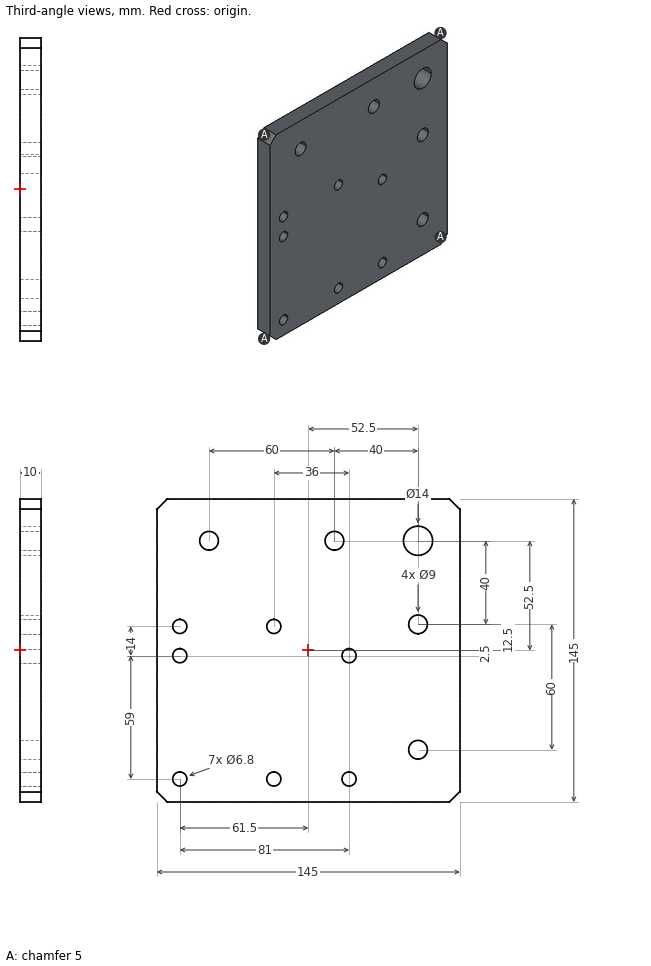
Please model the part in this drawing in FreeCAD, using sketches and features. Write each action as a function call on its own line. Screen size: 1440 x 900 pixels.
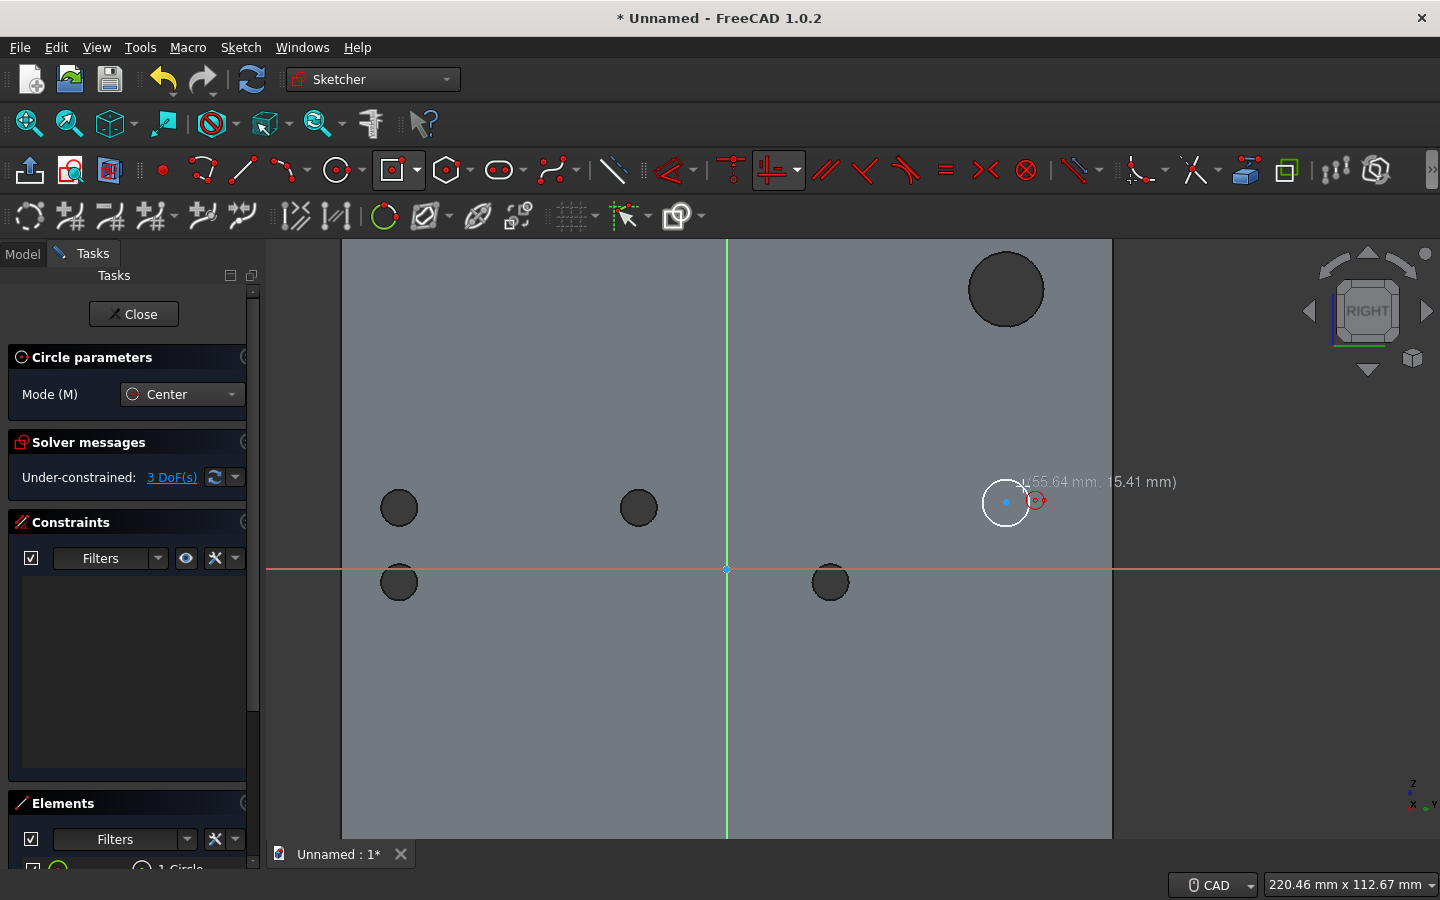
scroll(875, 505, down, 2)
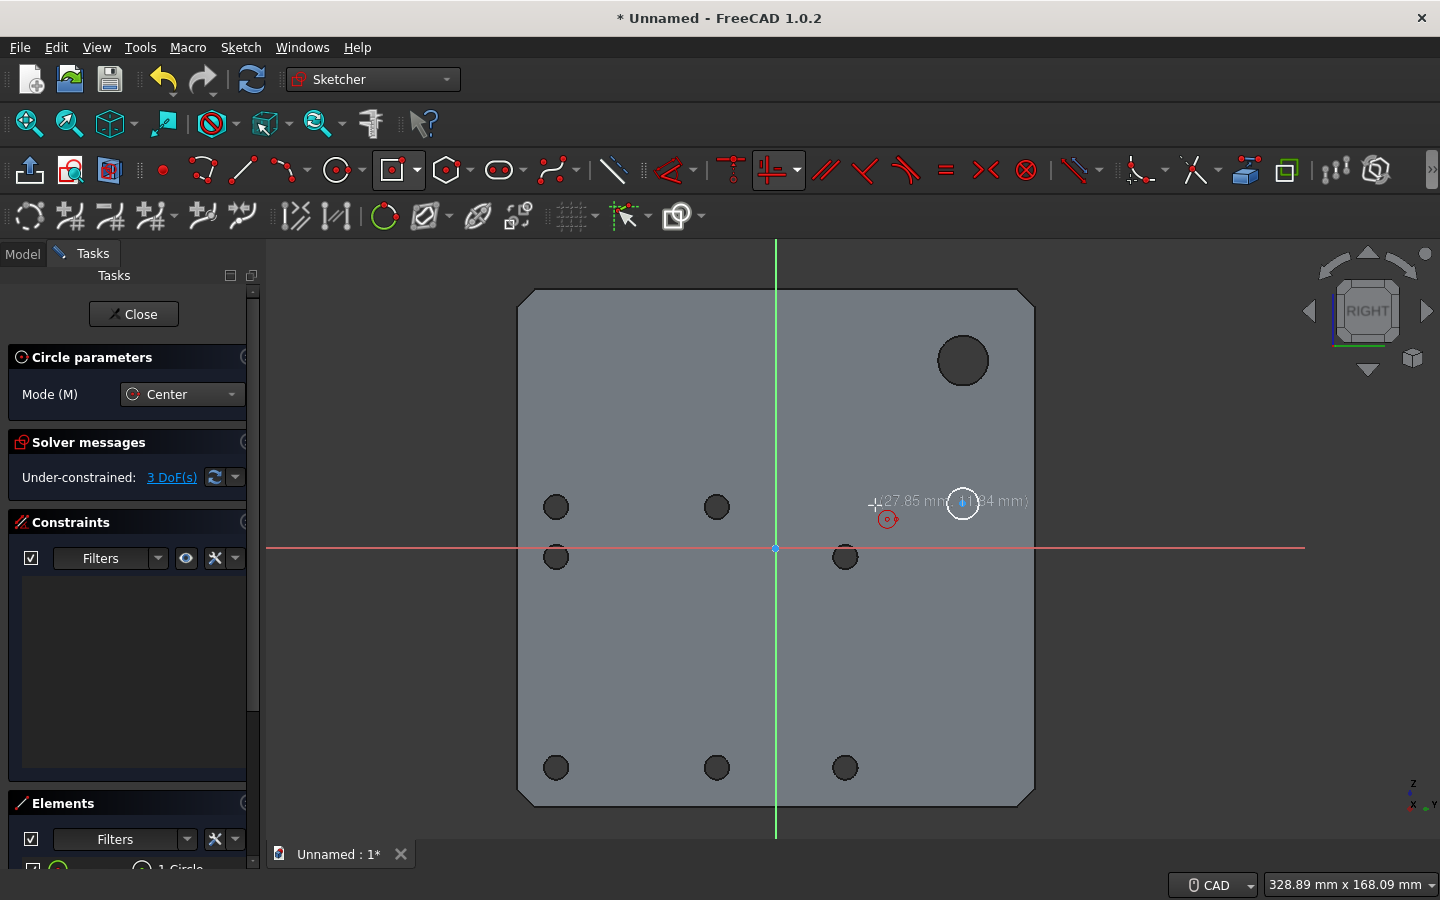
scroll(963, 718, up, 2)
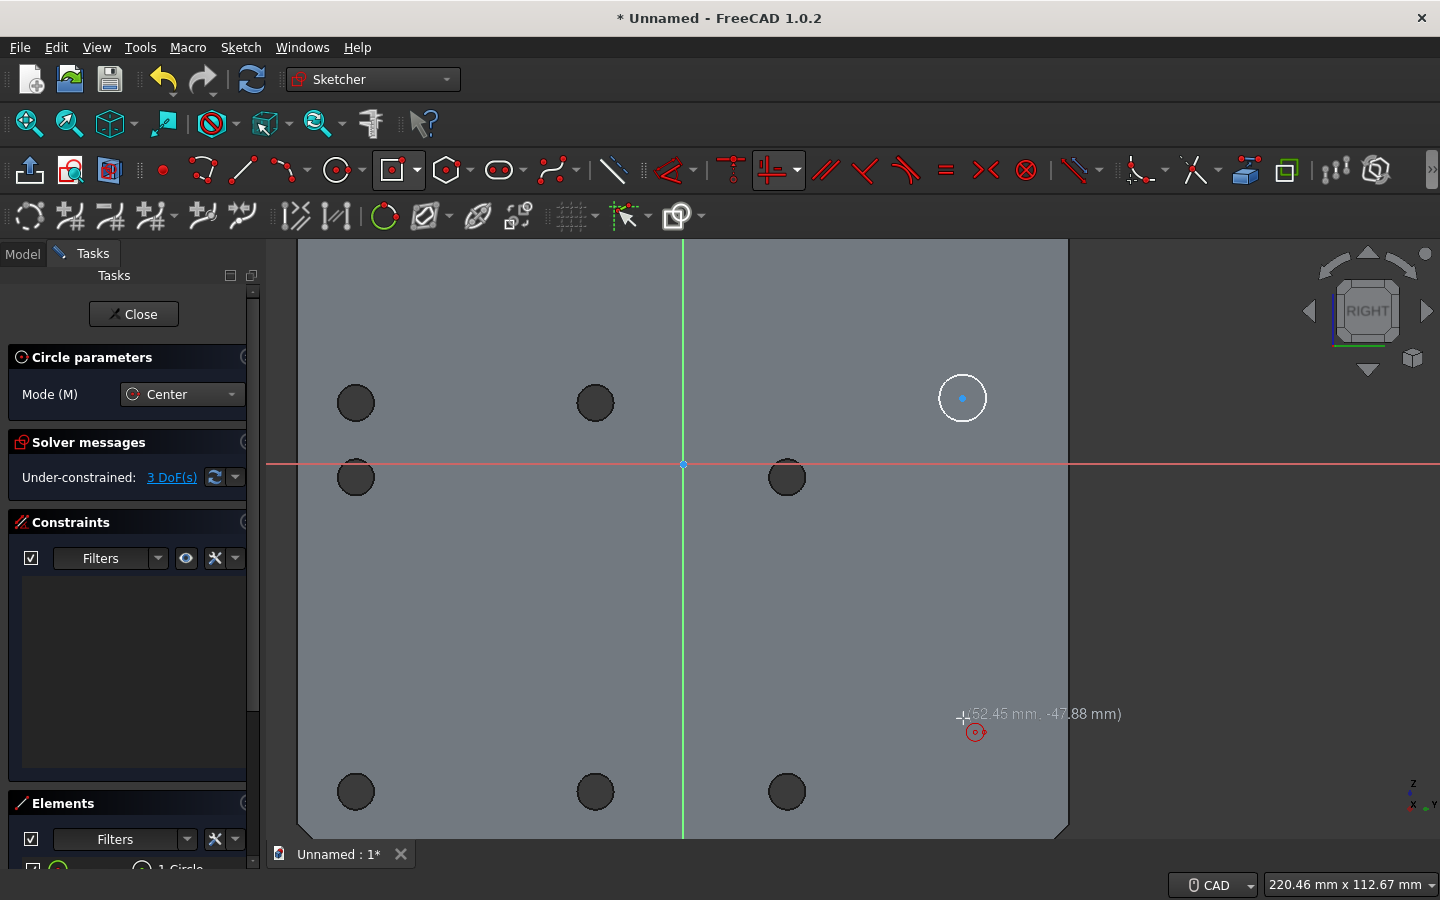
click(963, 717)
click(980, 700)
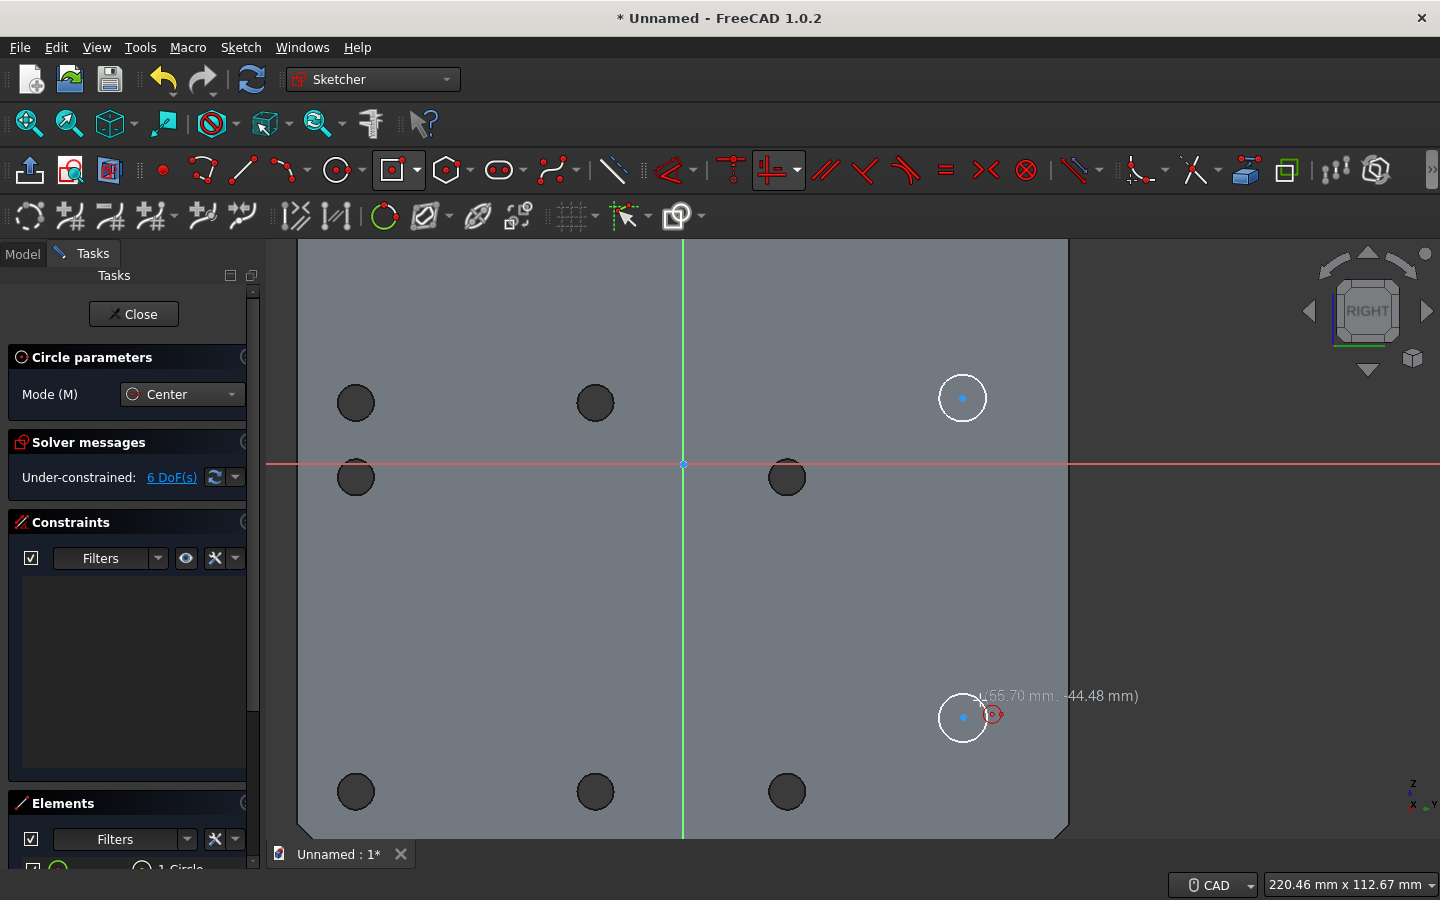
scroll(963, 718, down, 2)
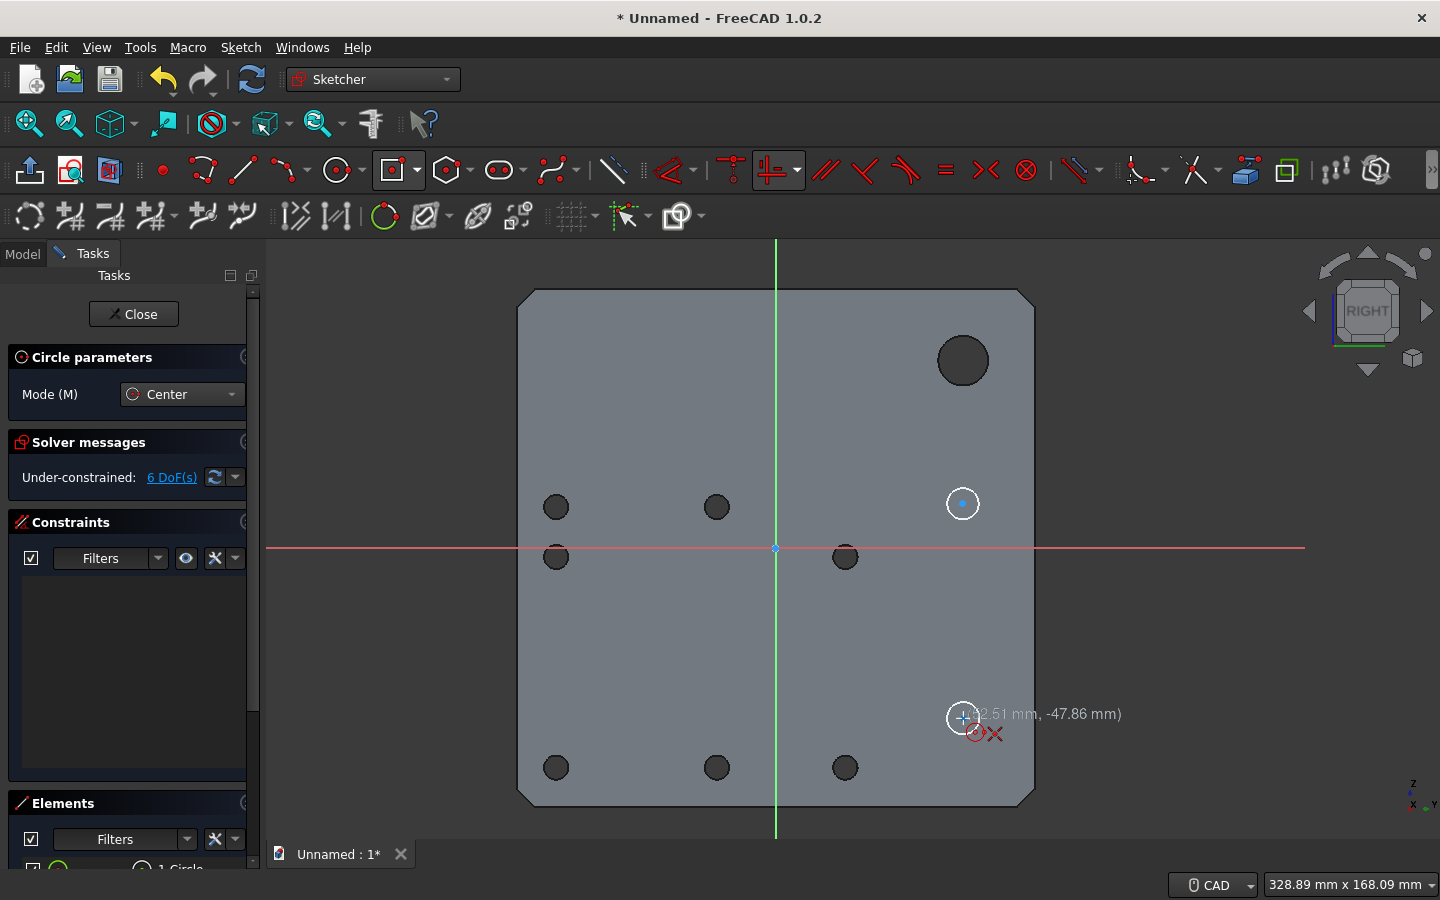
scroll(820, 361, up, 2)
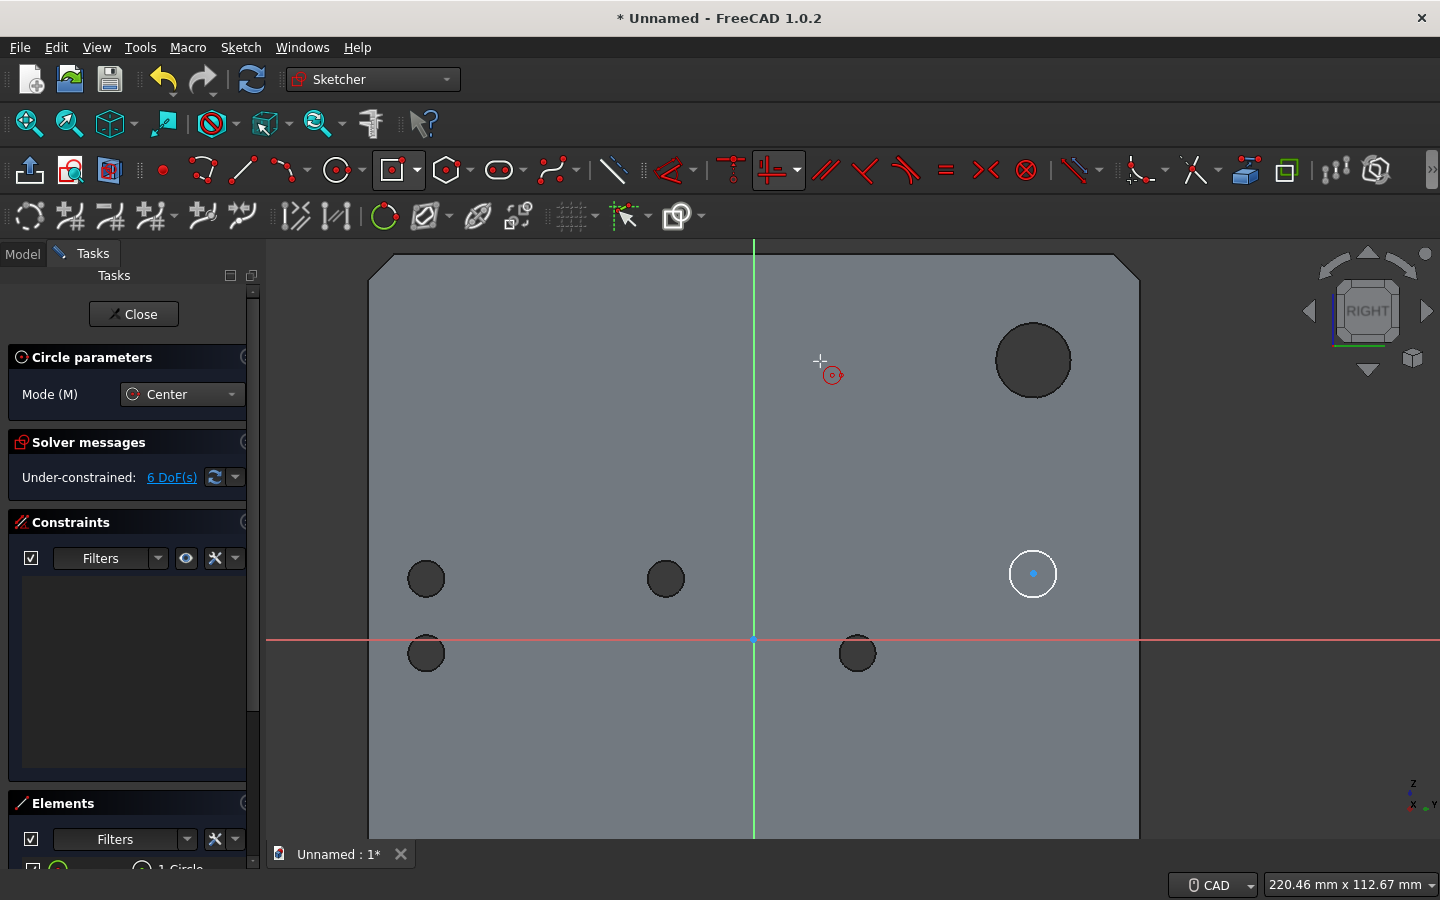
click(820, 360)
click(837, 343)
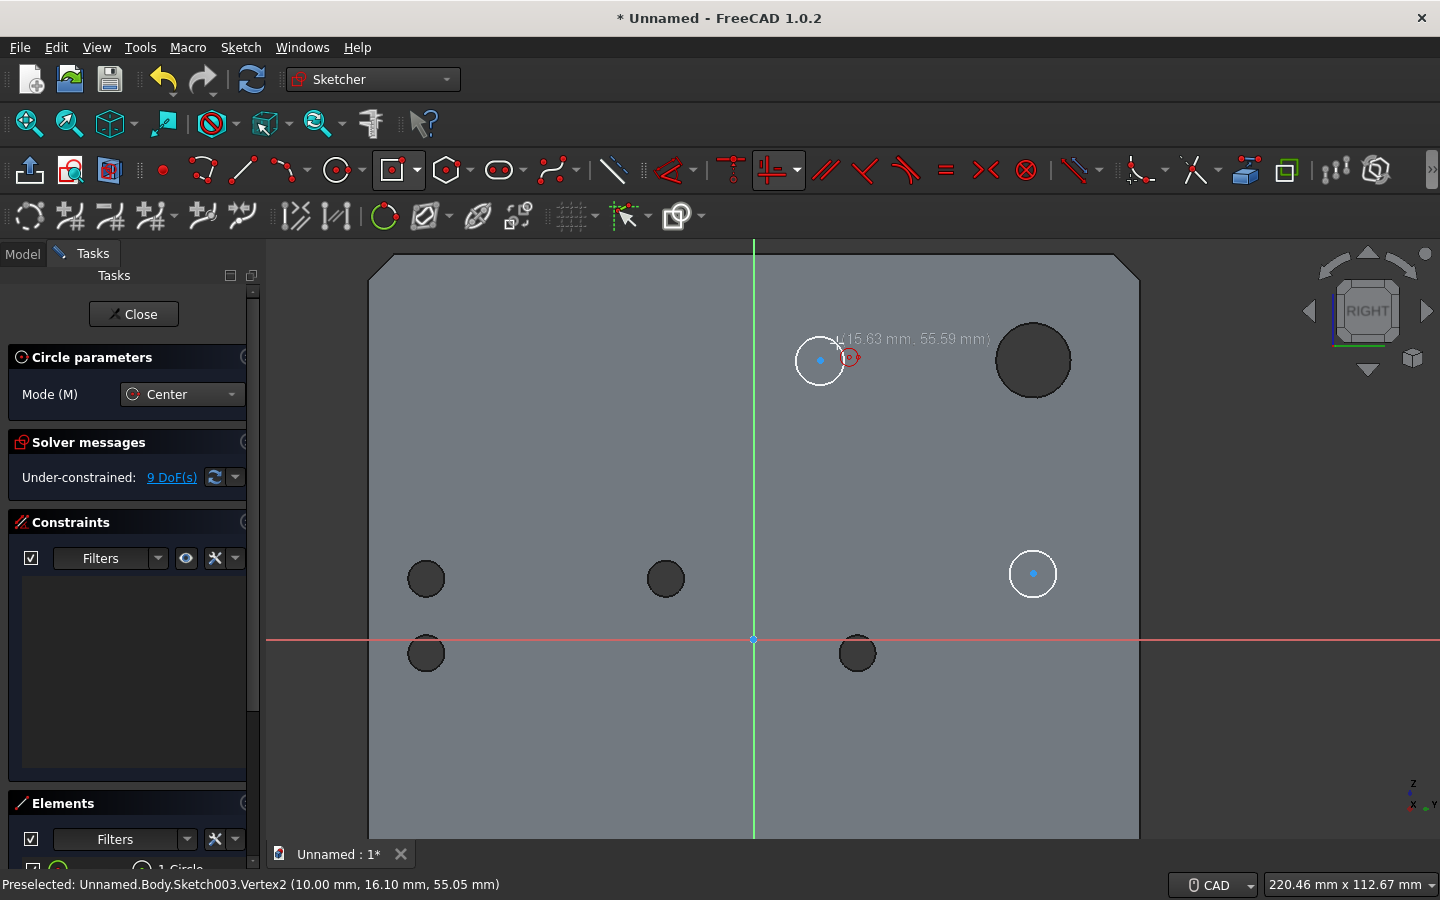
click(501, 360)
click(518, 343)
key(Escape)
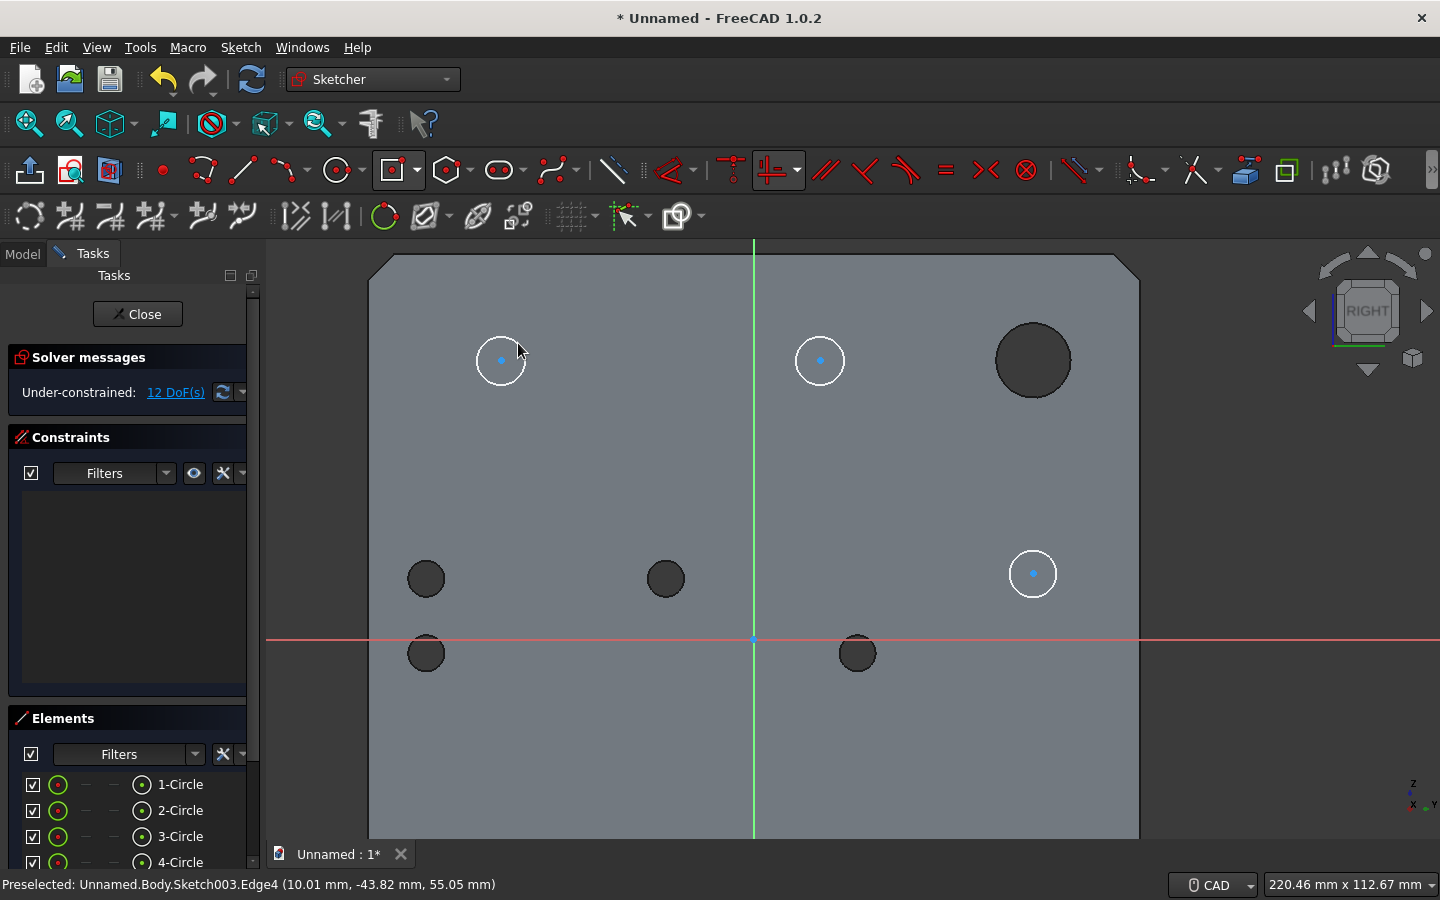
click(1050, 557)